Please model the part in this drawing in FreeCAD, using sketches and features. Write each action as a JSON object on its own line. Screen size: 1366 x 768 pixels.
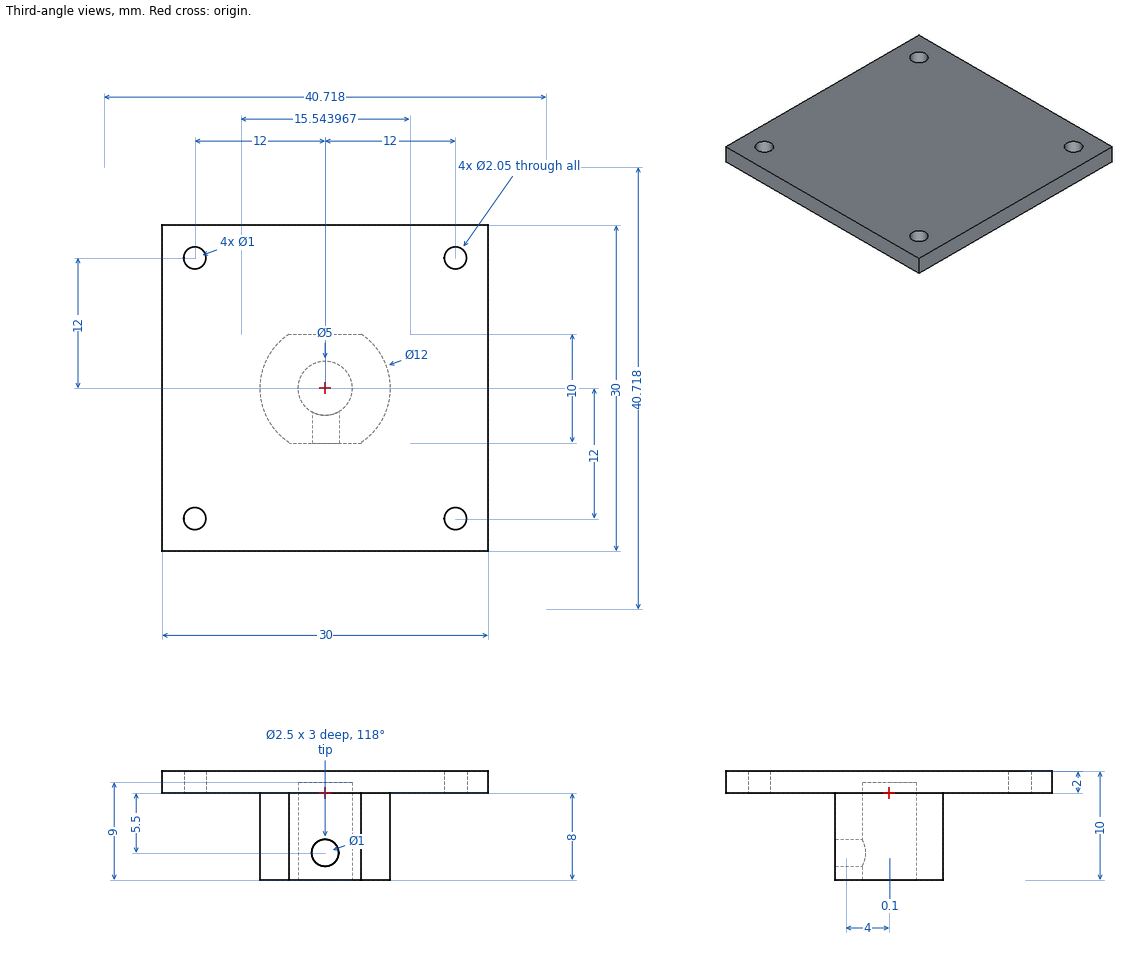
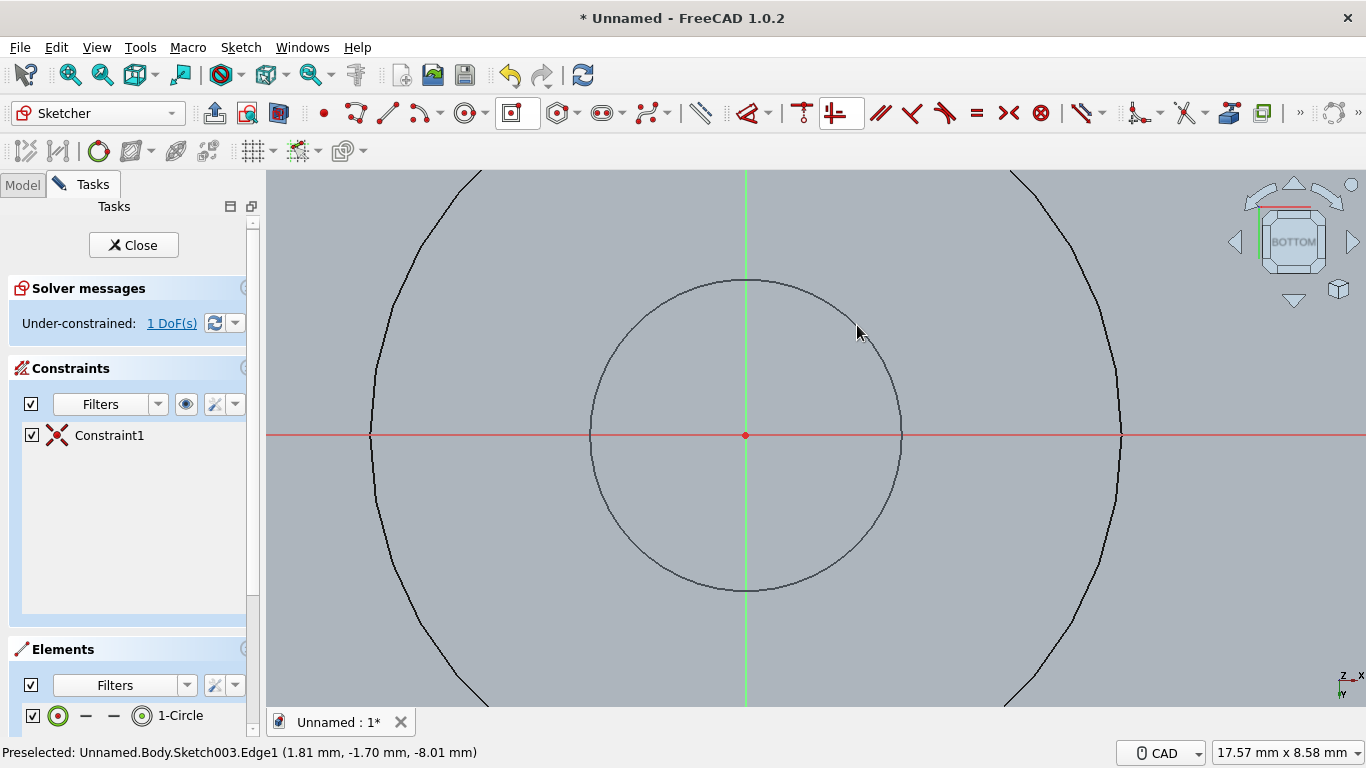
{"action": "key", "text": "d"}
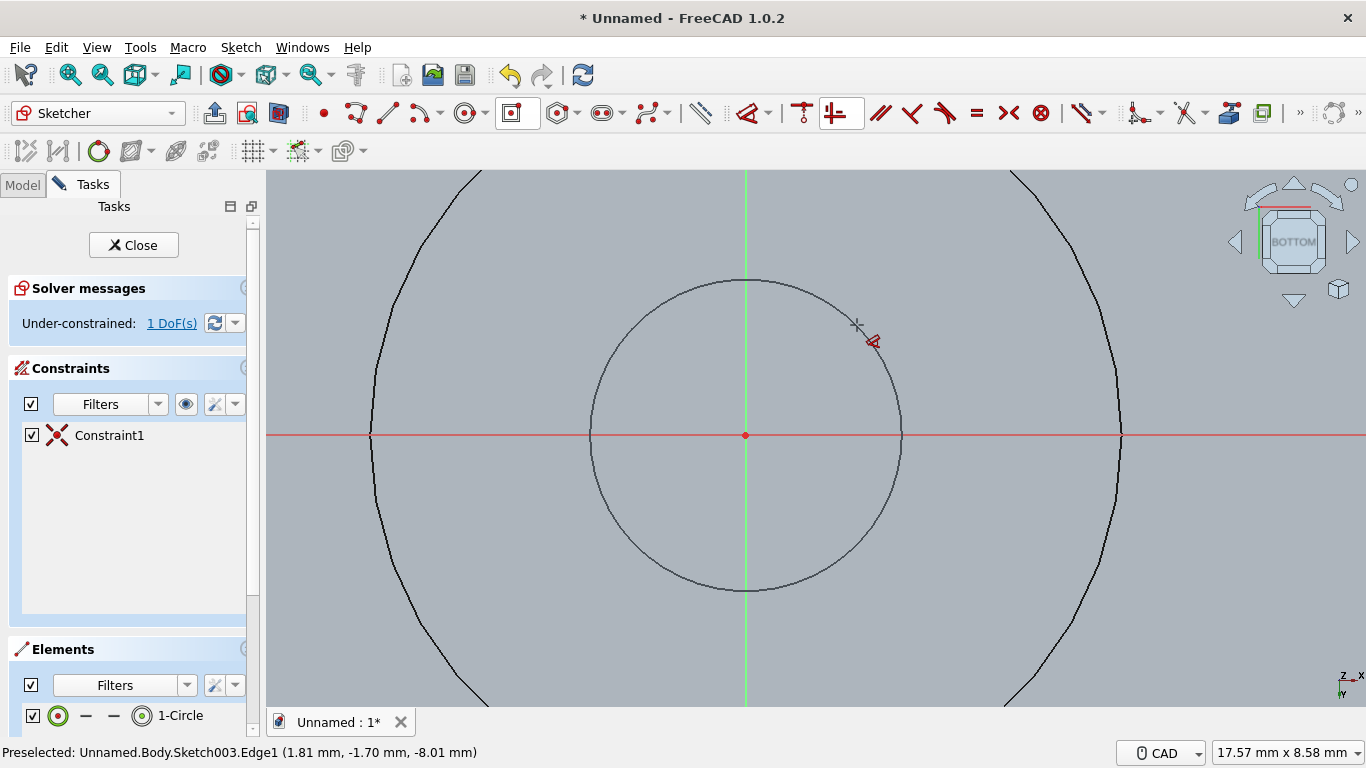
{"action": "left_click", "coordinate": [856, 325]}
{"action": "left_click", "coordinate": [879, 302]}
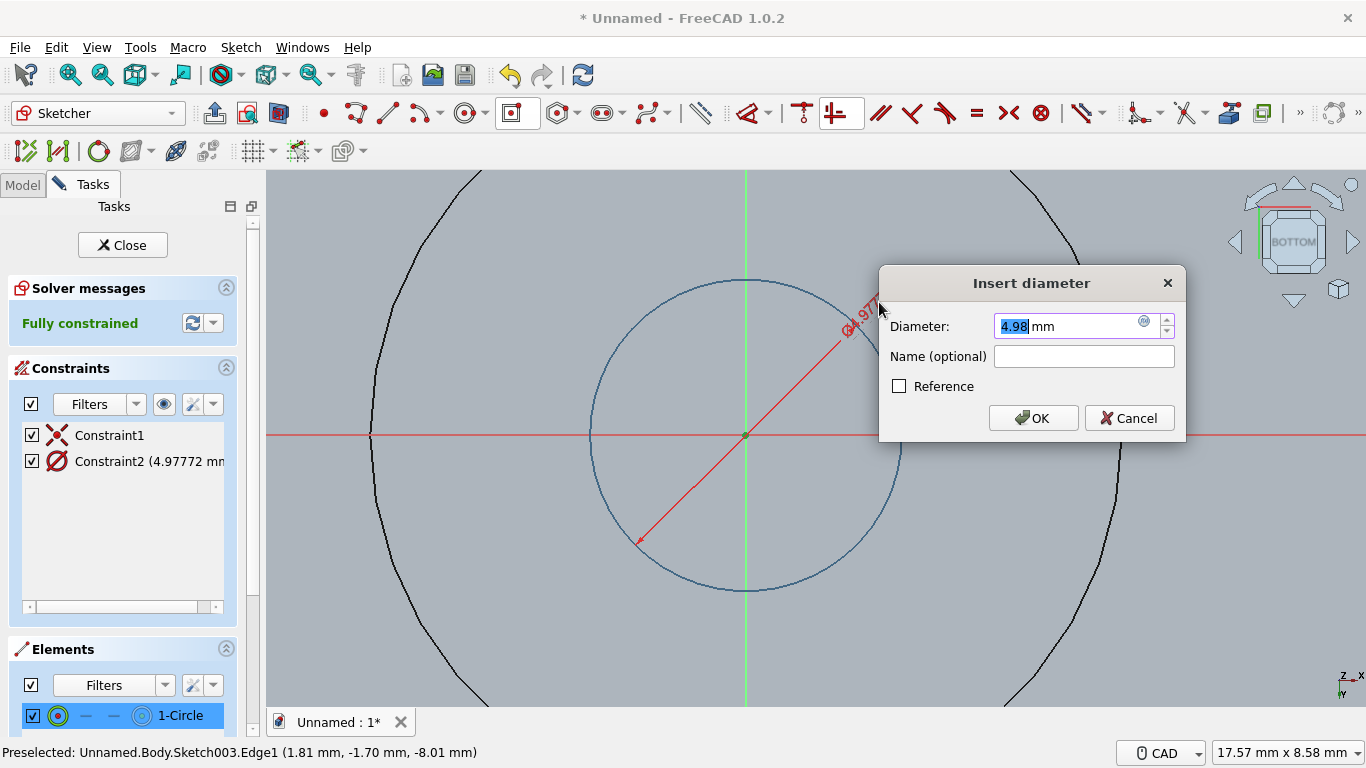
{"action": "type", "text": "5"}
{"action": "key", "text": "Return"}
{"action": "key", "text": "Escape"}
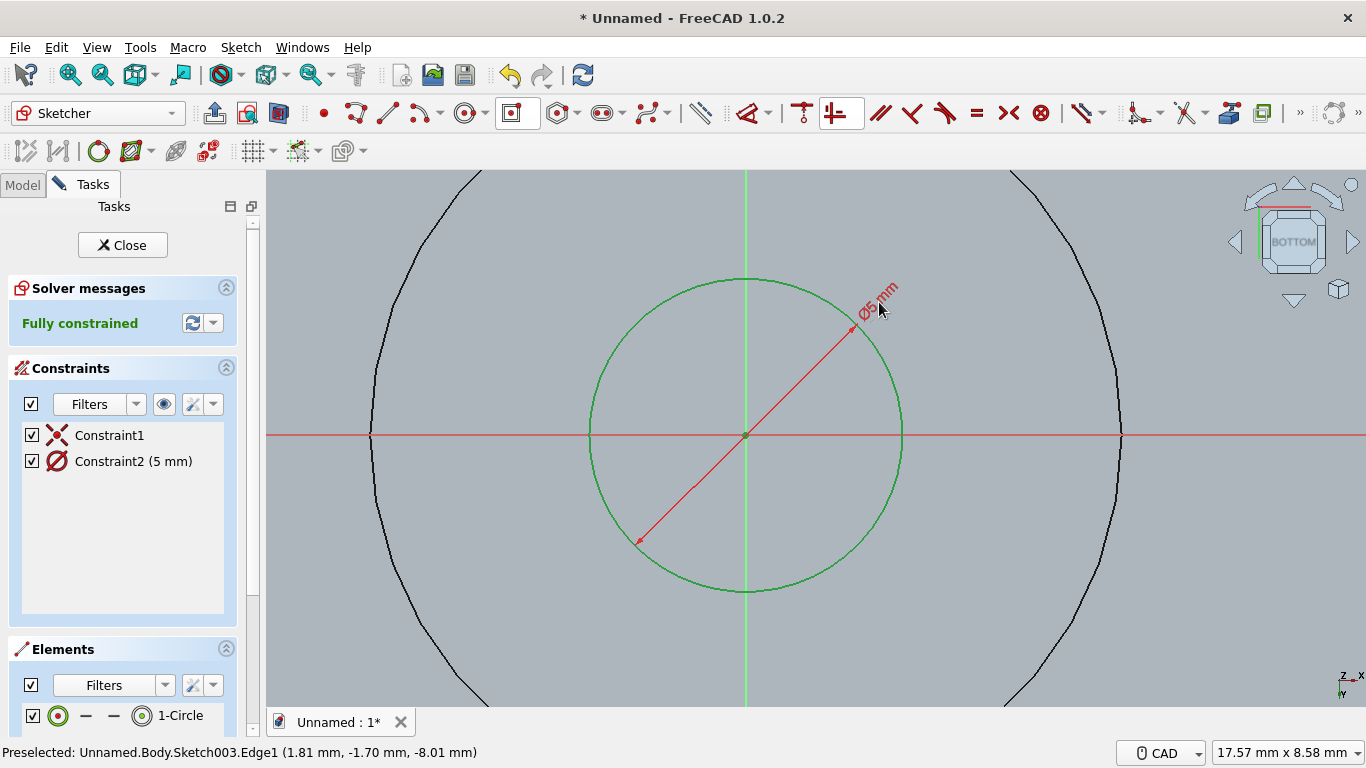
{"action": "left_click", "coordinate": [123, 245]}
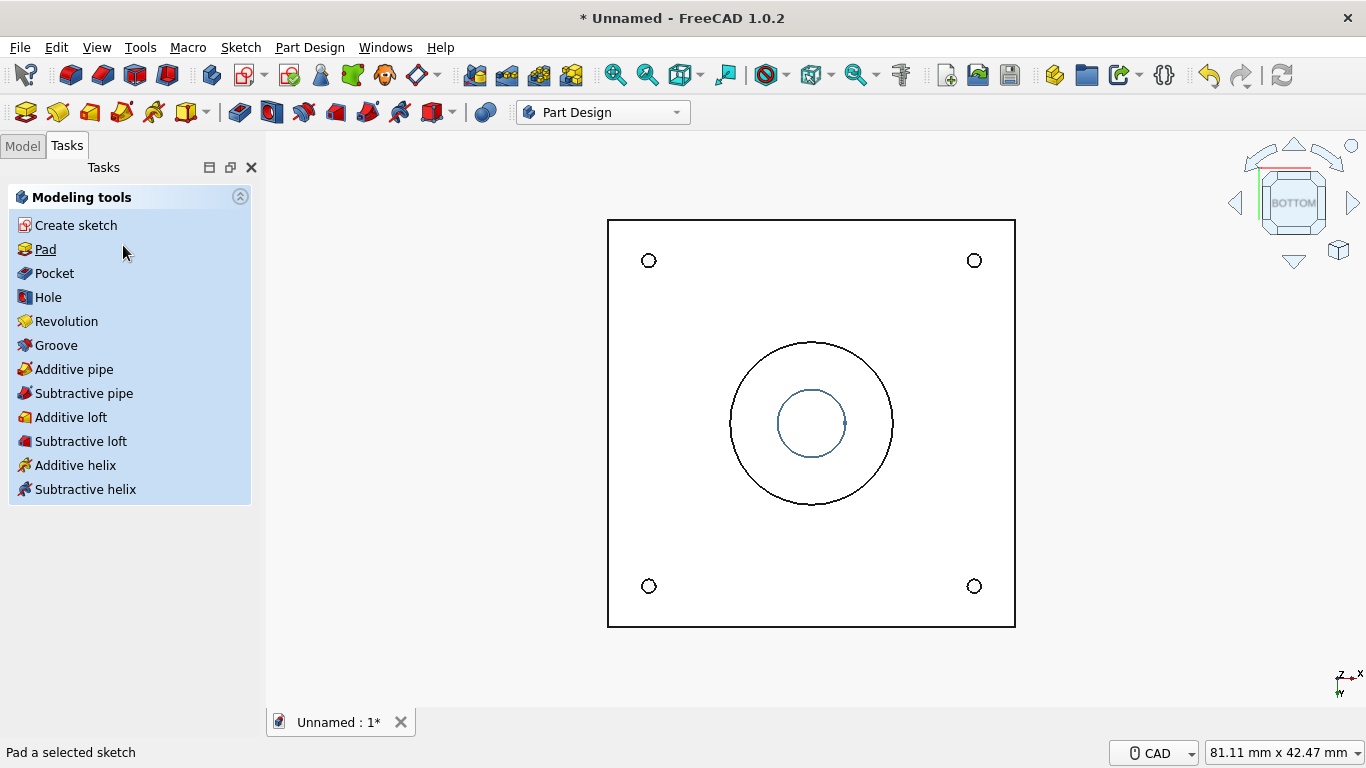
{"action": "left_click", "coordinate": [240, 112]}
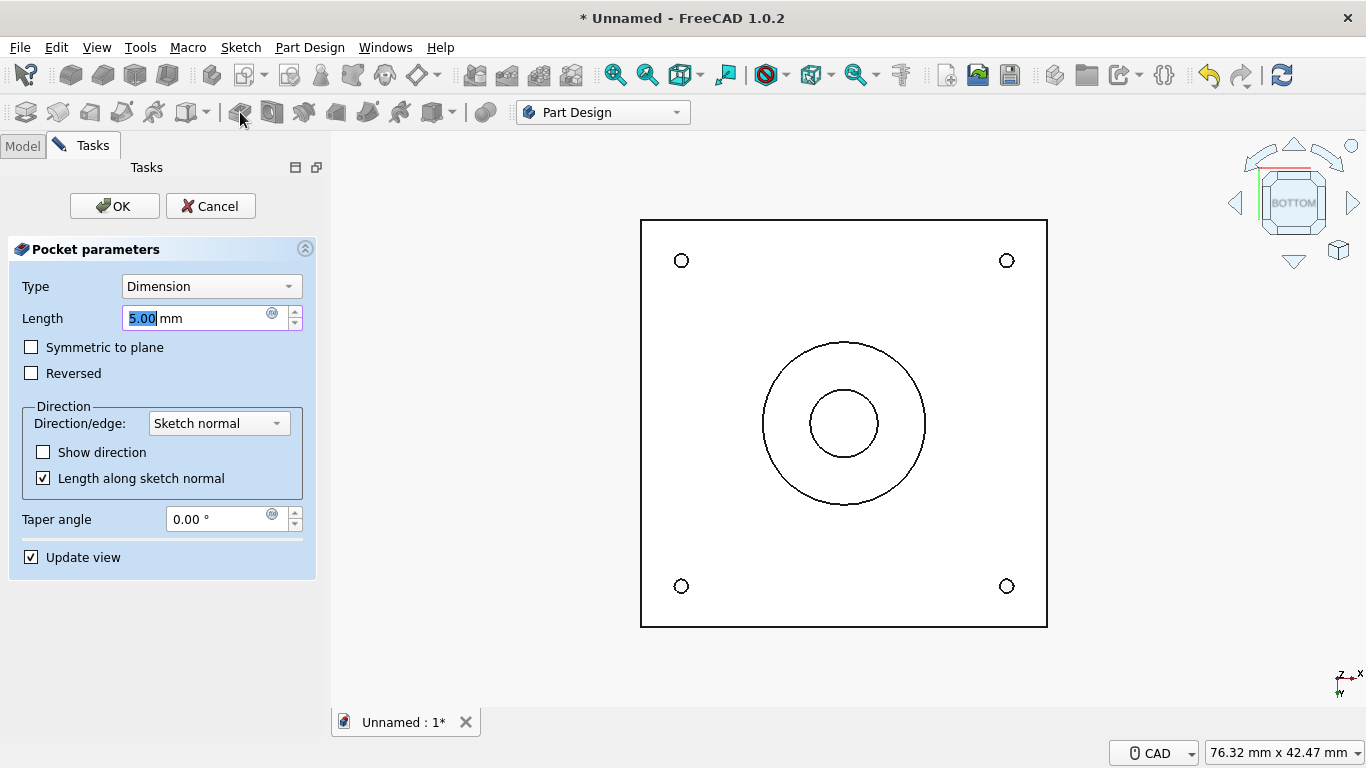
{"action": "type", "text": "9"}
{"action": "key", "text": "Tab"}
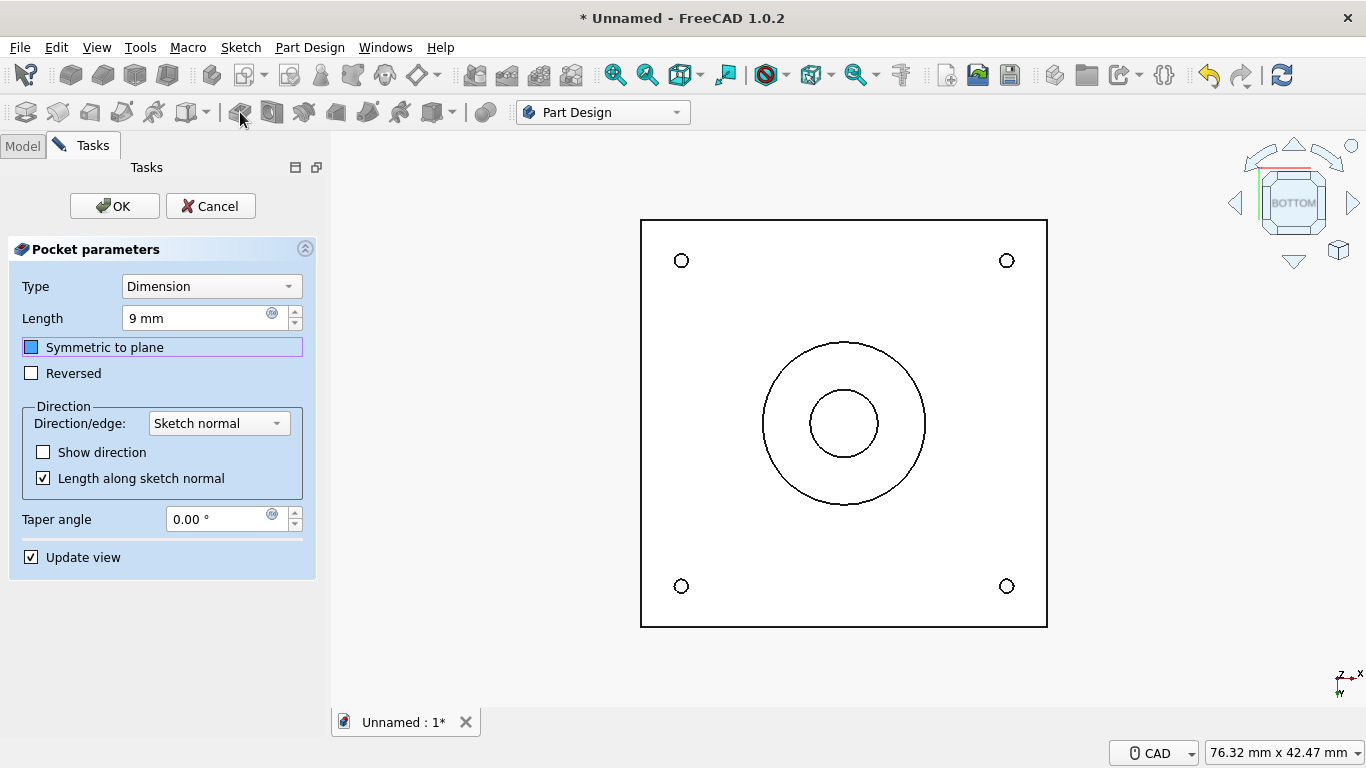
{"action": "left_click", "coordinate": [115, 206]}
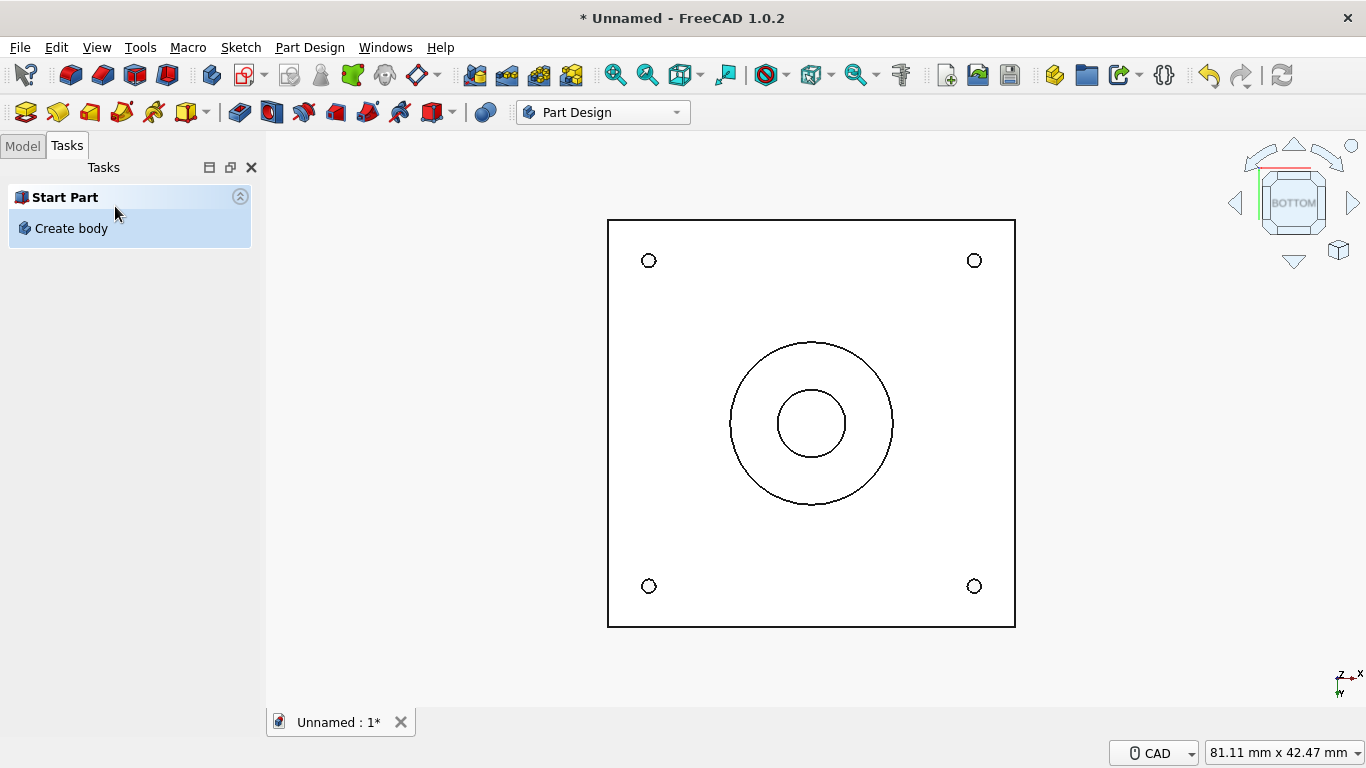
{"action": "left_click", "coordinate": [244, 76]}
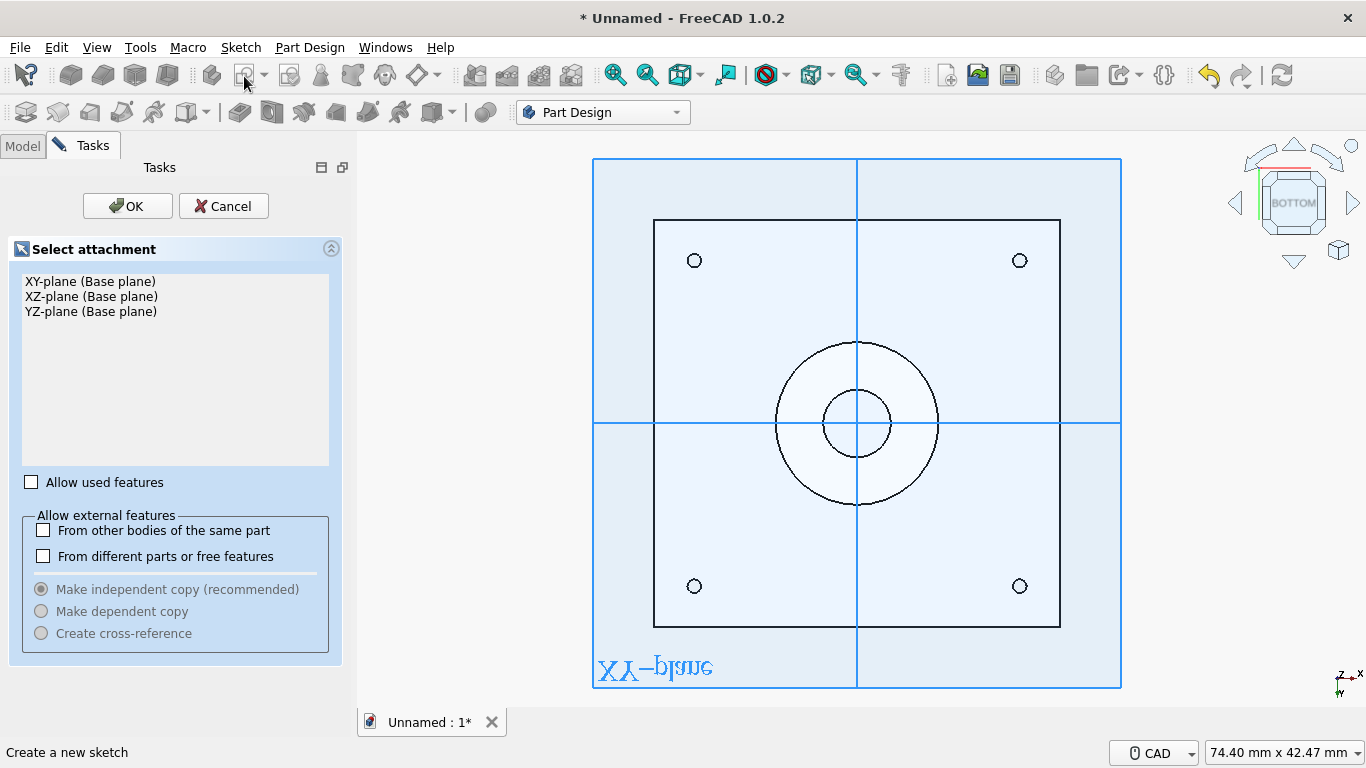
{"action": "left_click", "coordinate": [82, 296]}